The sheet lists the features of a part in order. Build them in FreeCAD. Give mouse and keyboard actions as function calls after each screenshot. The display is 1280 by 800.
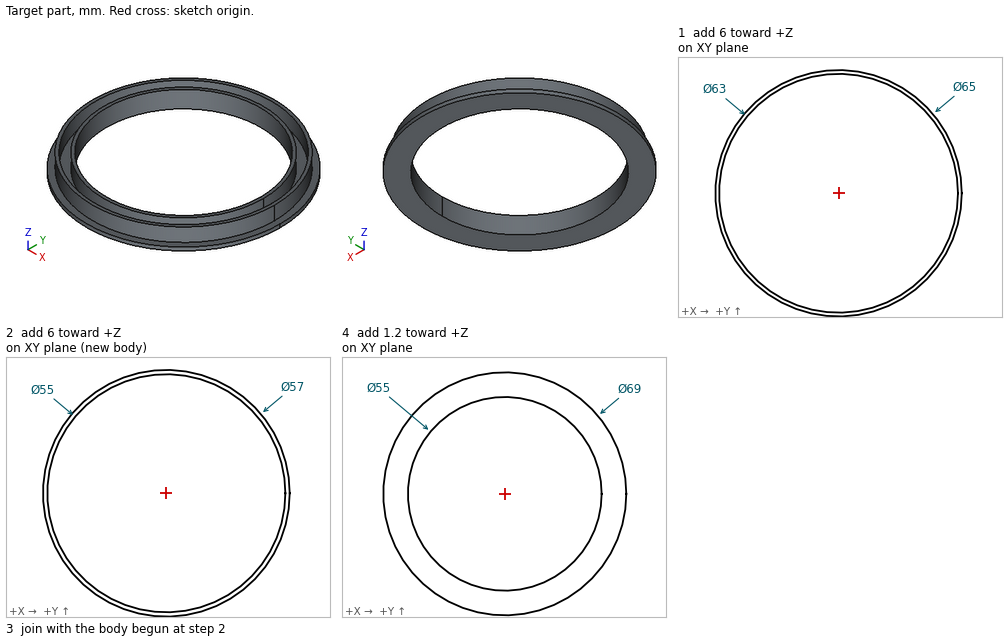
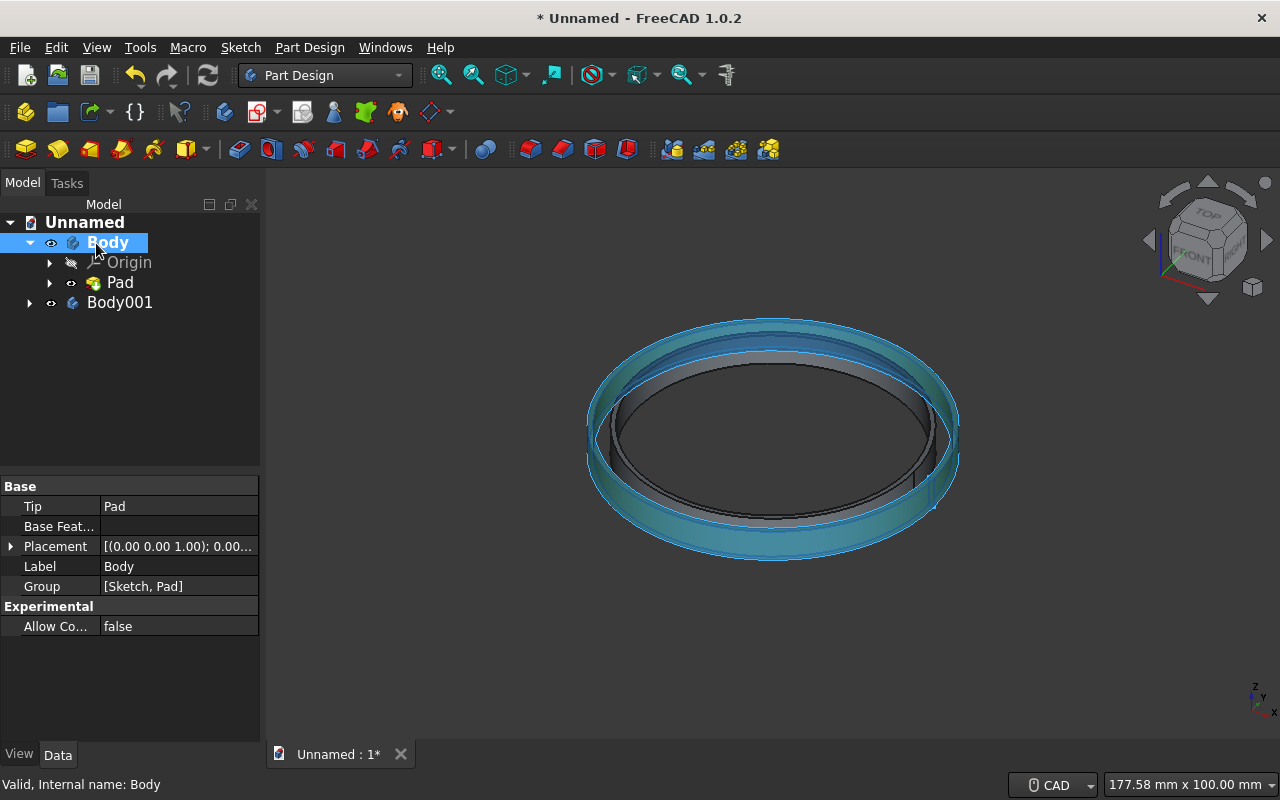
click(96, 243)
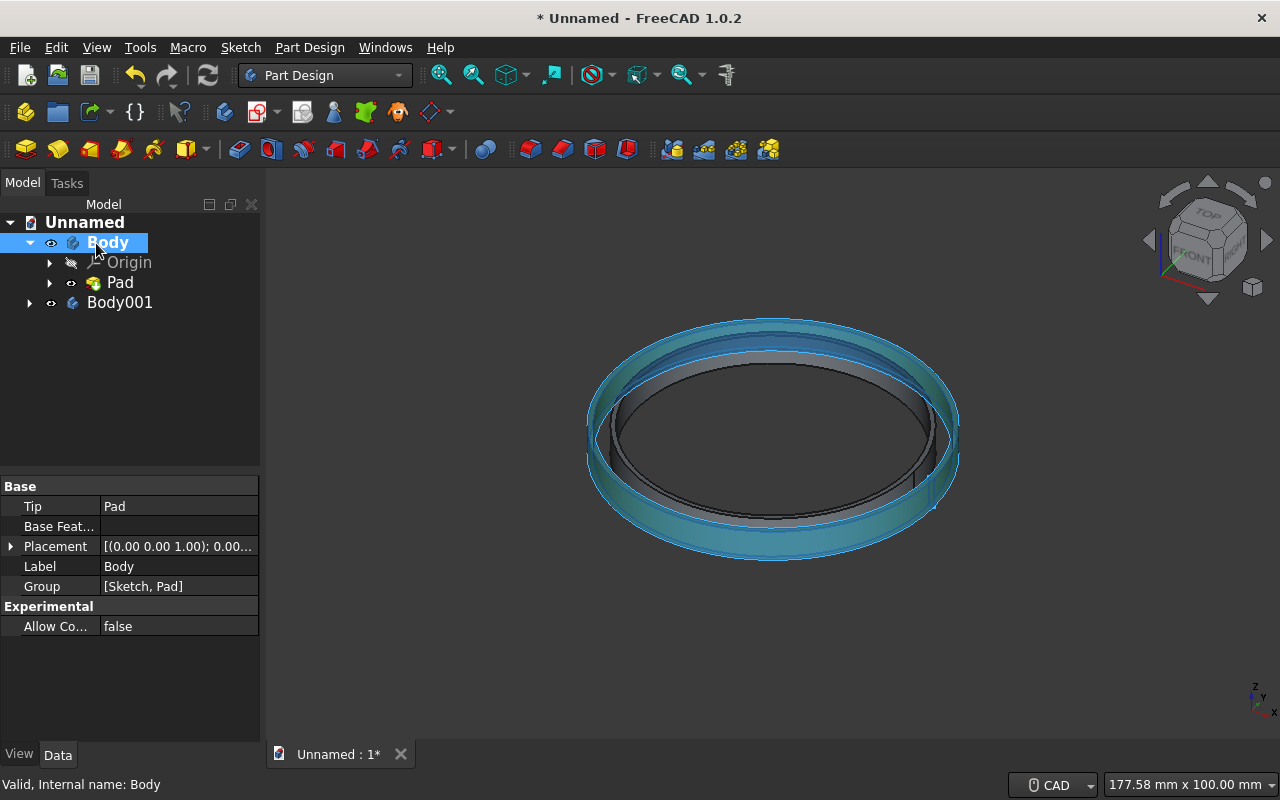
click(146, 626)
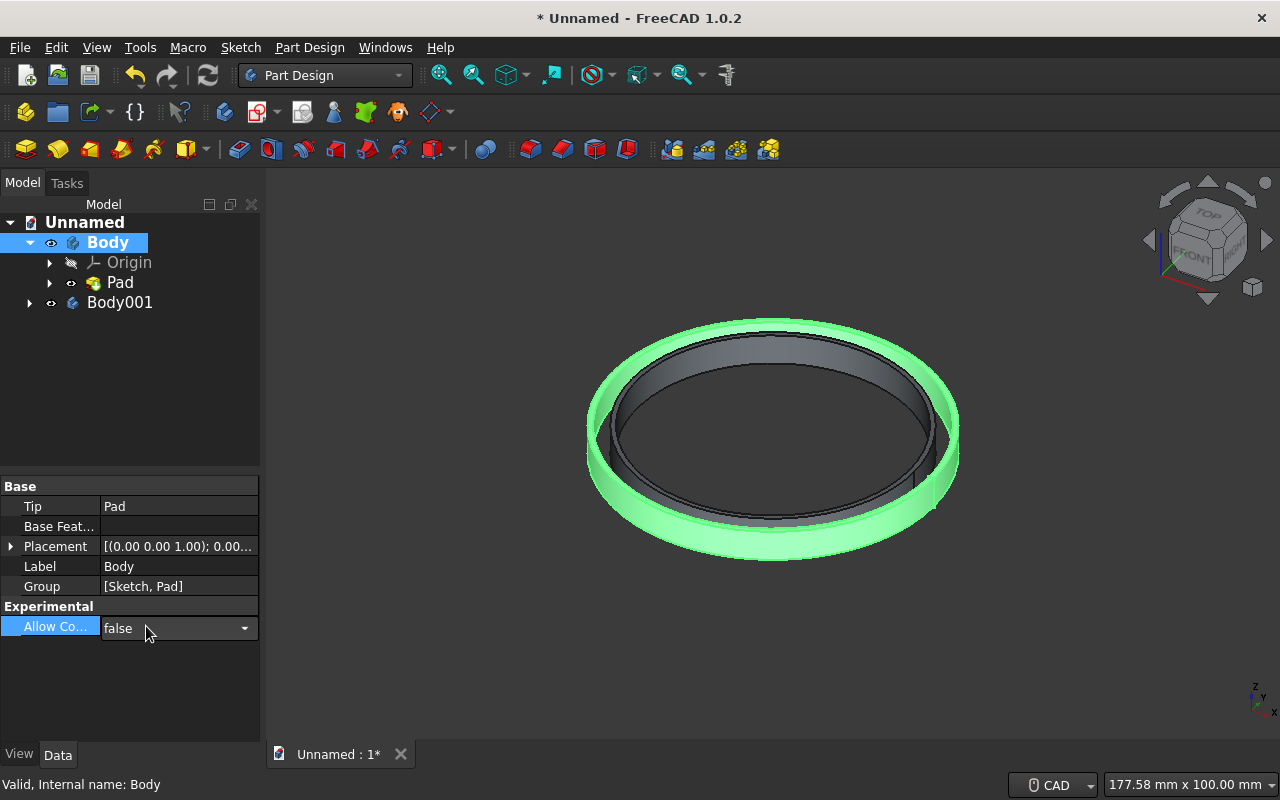
click(146, 626)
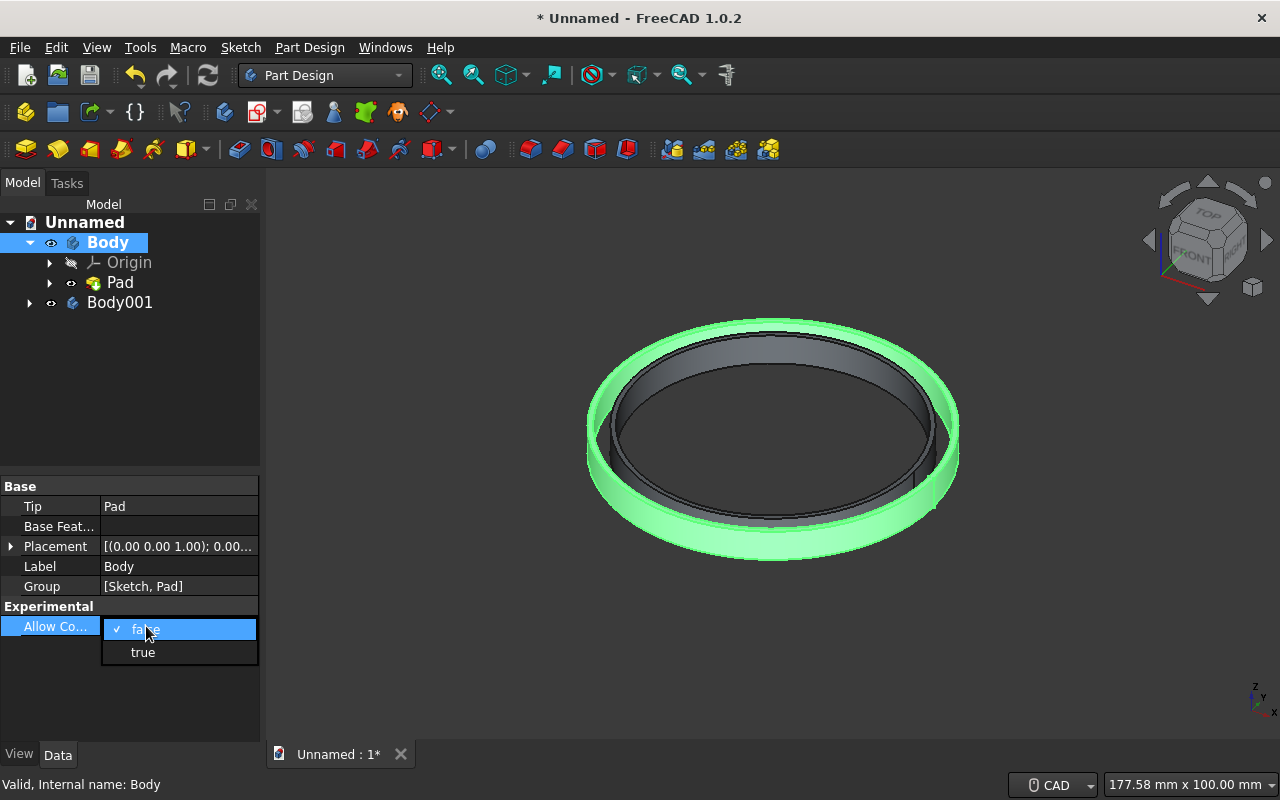
click(179, 652)
key(Return)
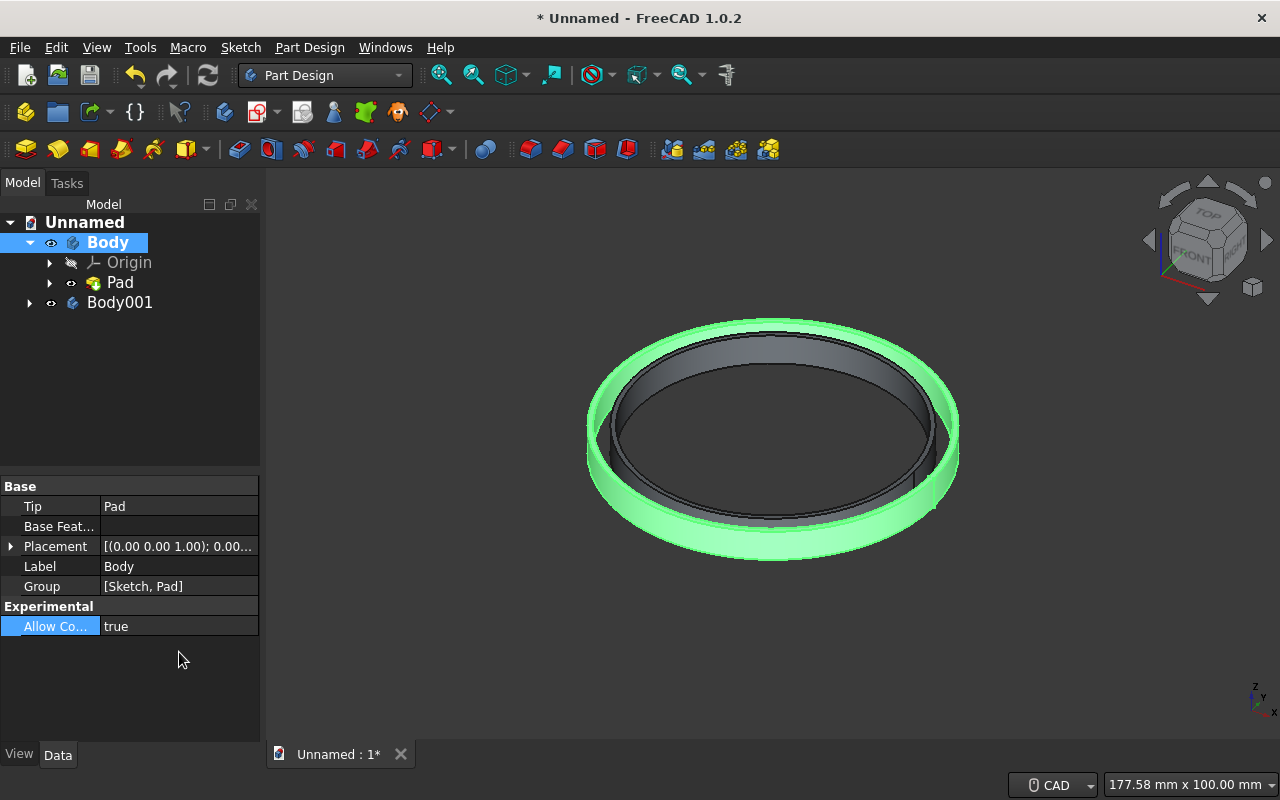
click(96, 303)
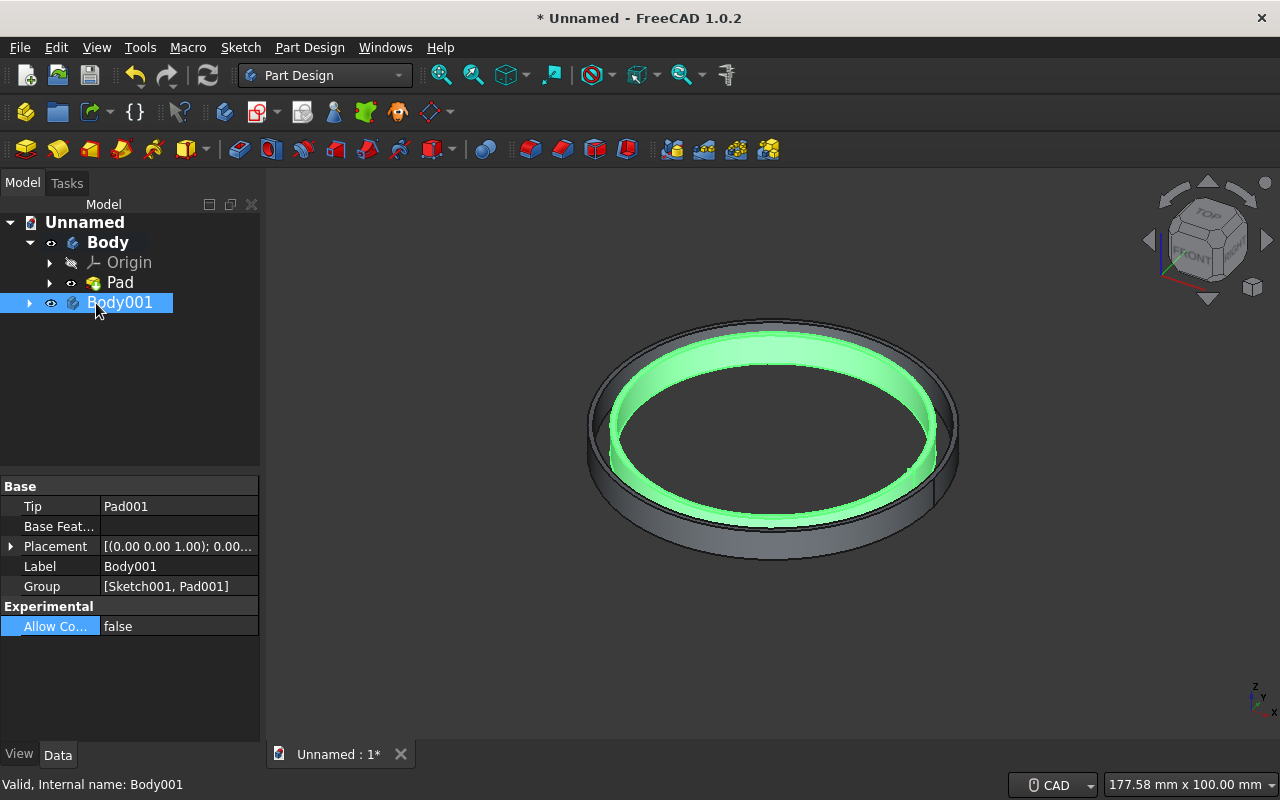
click(486, 150)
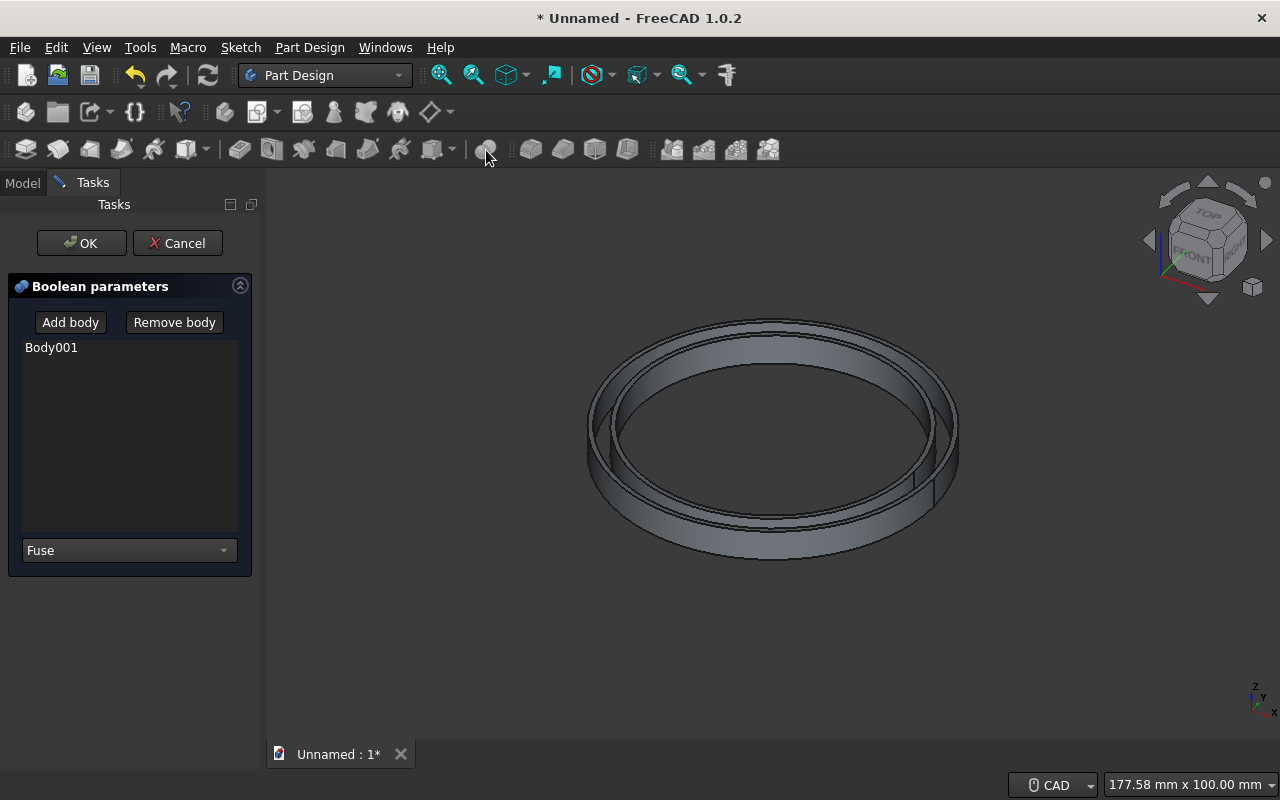
click(82, 243)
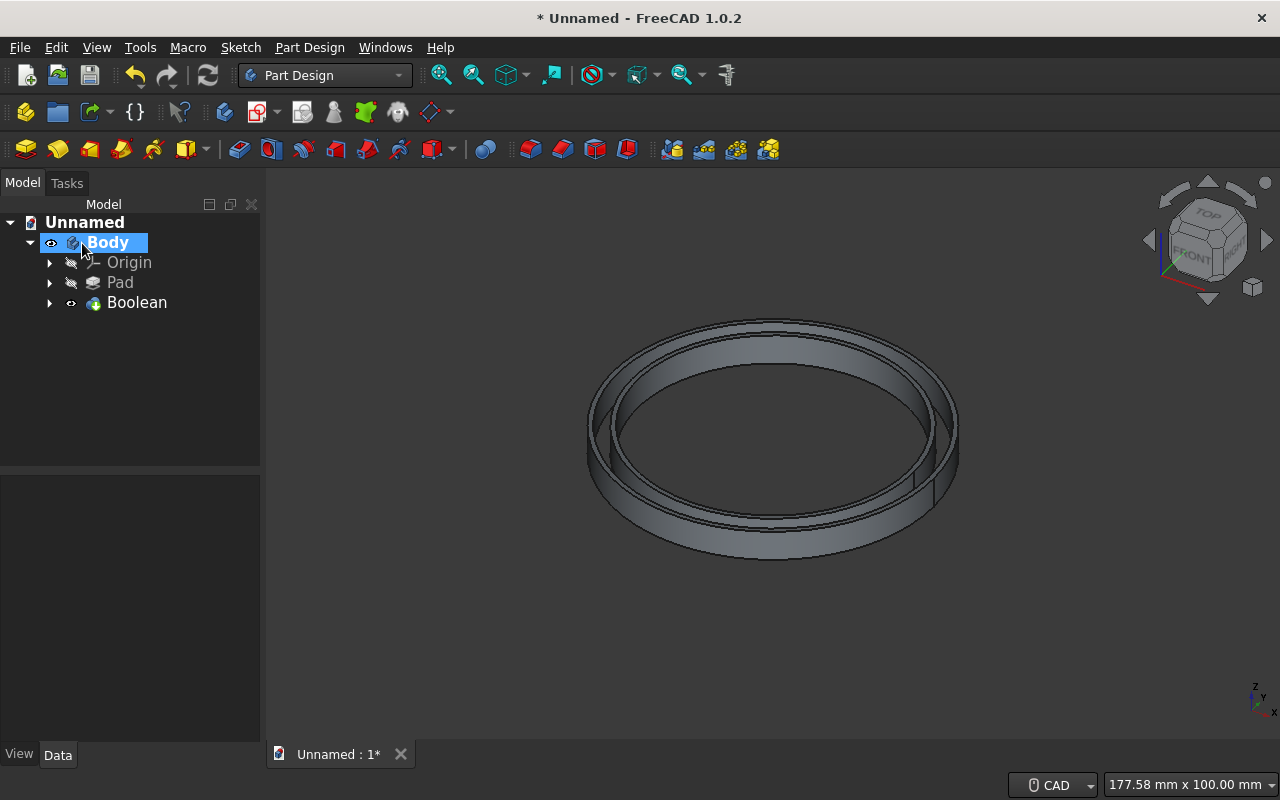
click(258, 112)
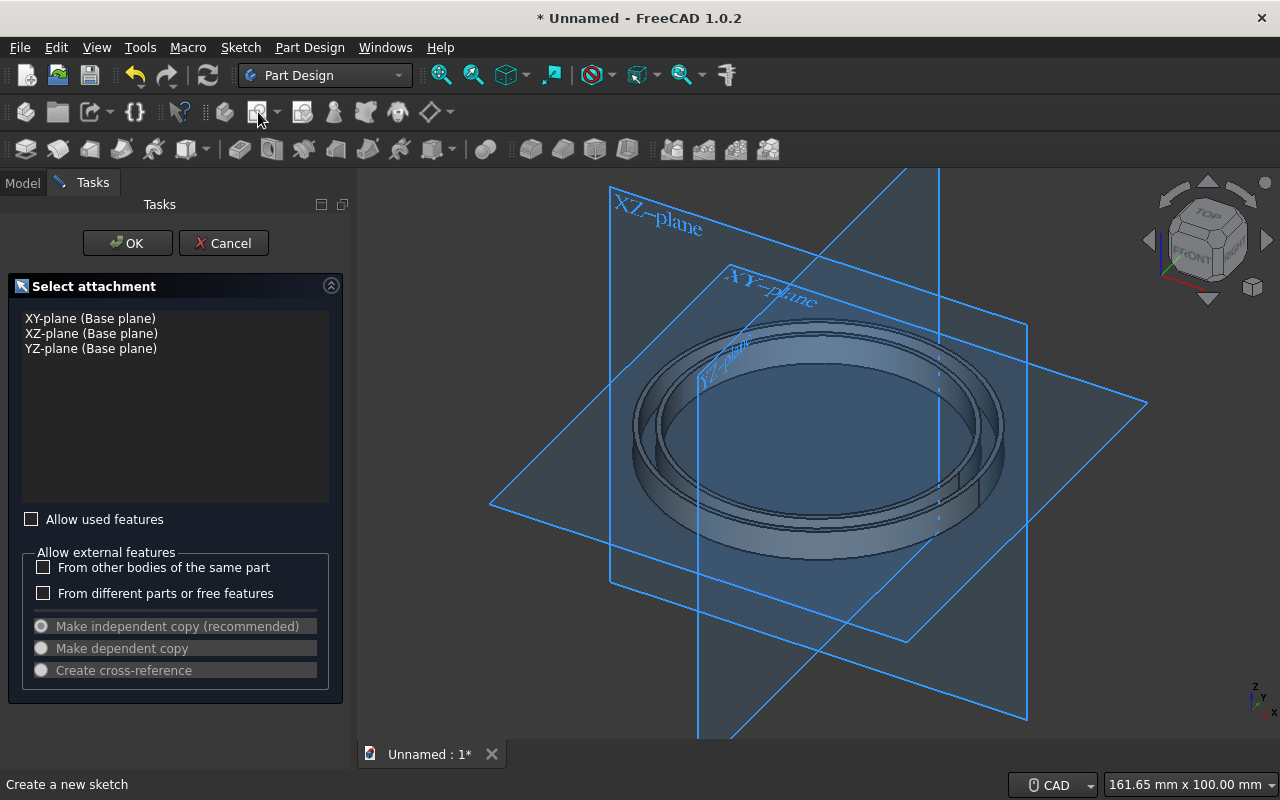
click(82, 318)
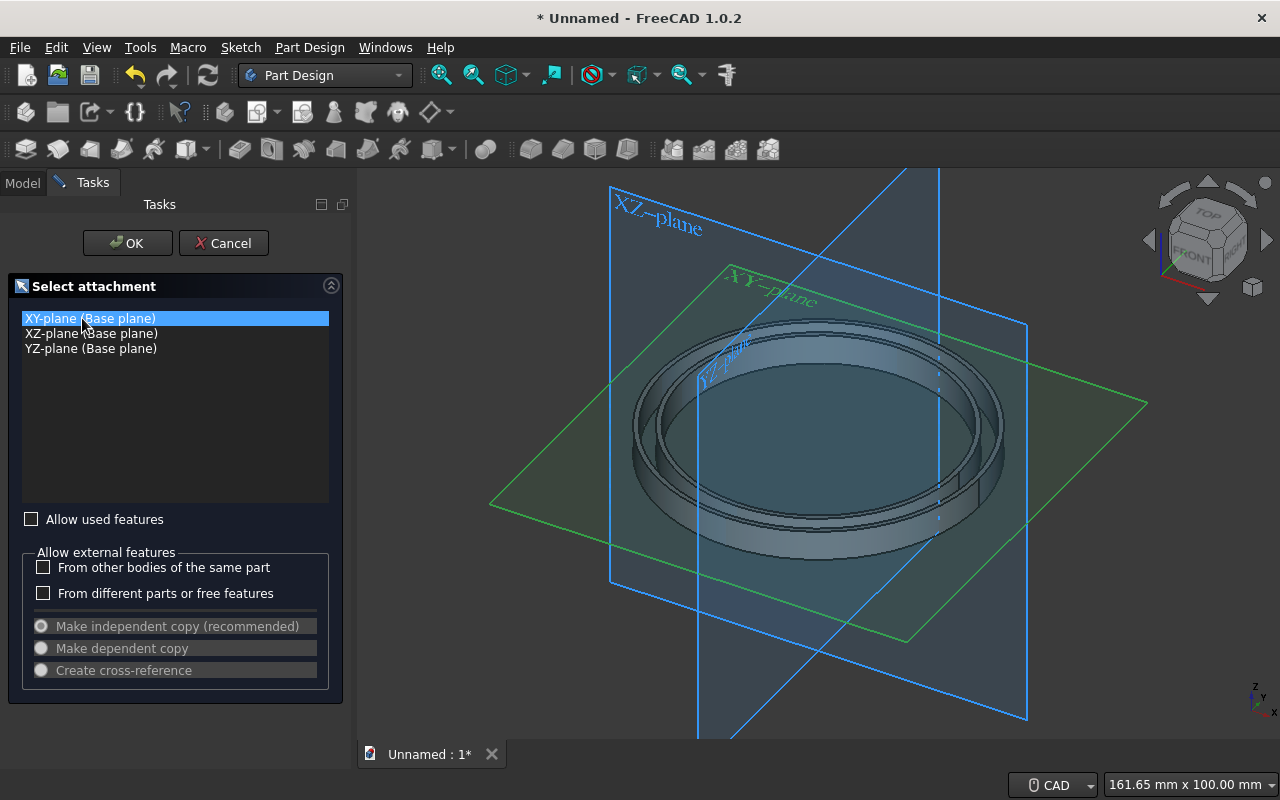
click(128, 243)